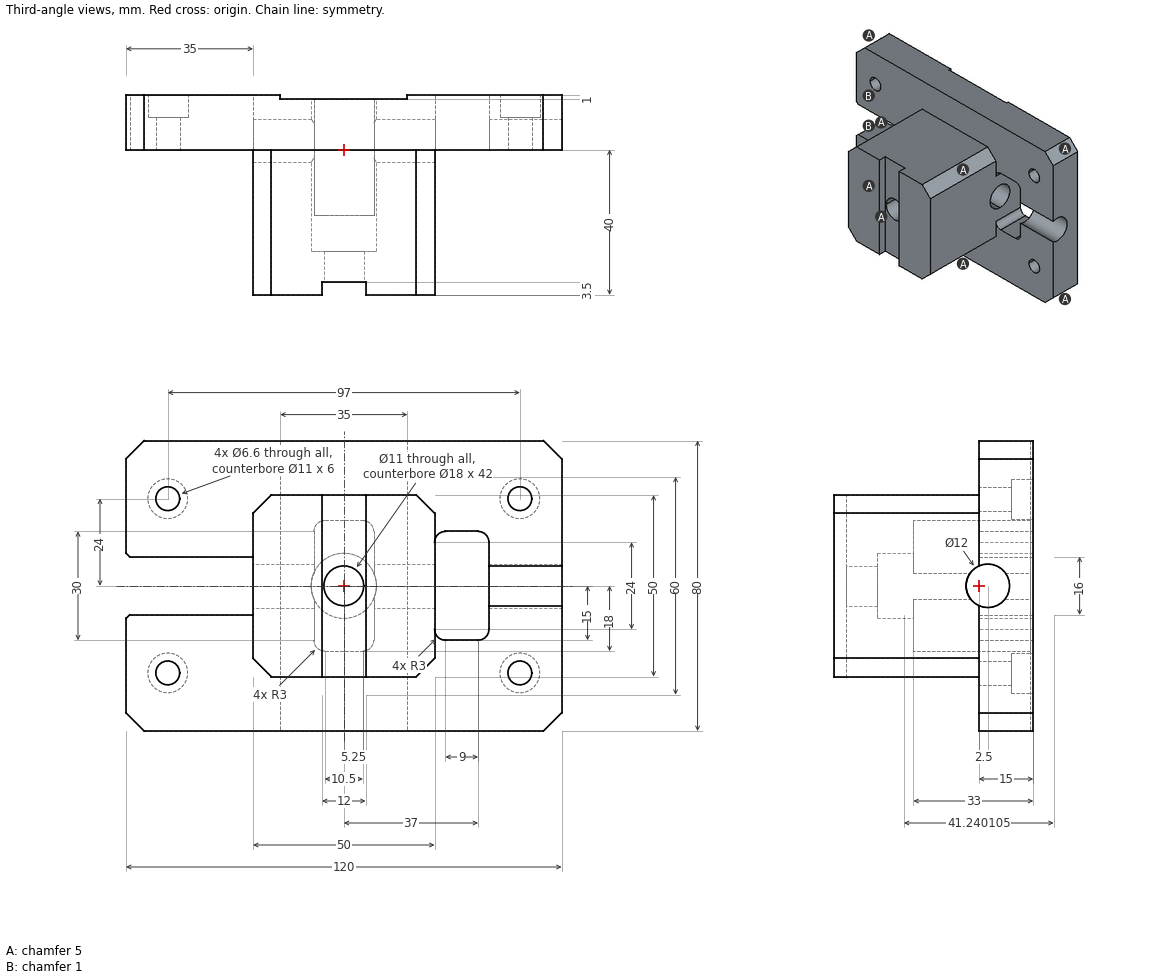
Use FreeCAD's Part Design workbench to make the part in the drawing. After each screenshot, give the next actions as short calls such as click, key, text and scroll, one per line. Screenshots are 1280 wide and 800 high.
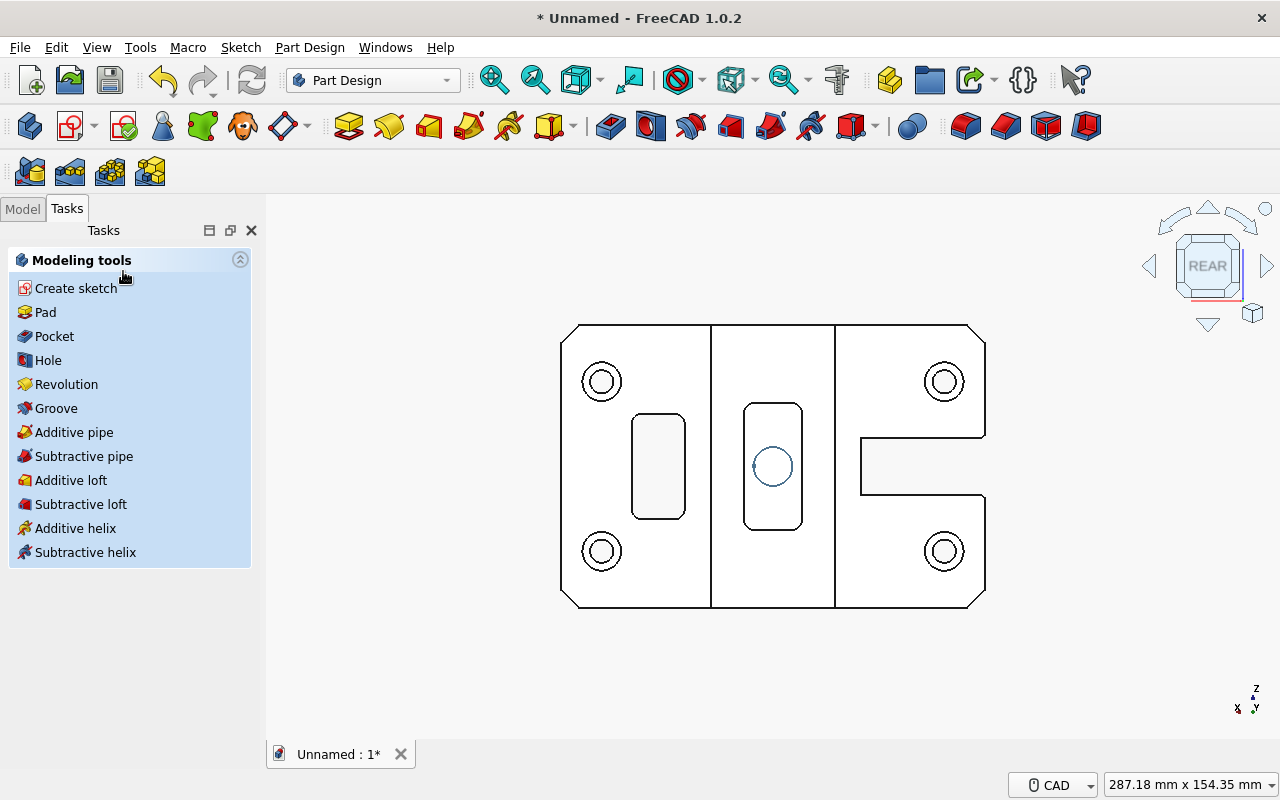
click(652, 126)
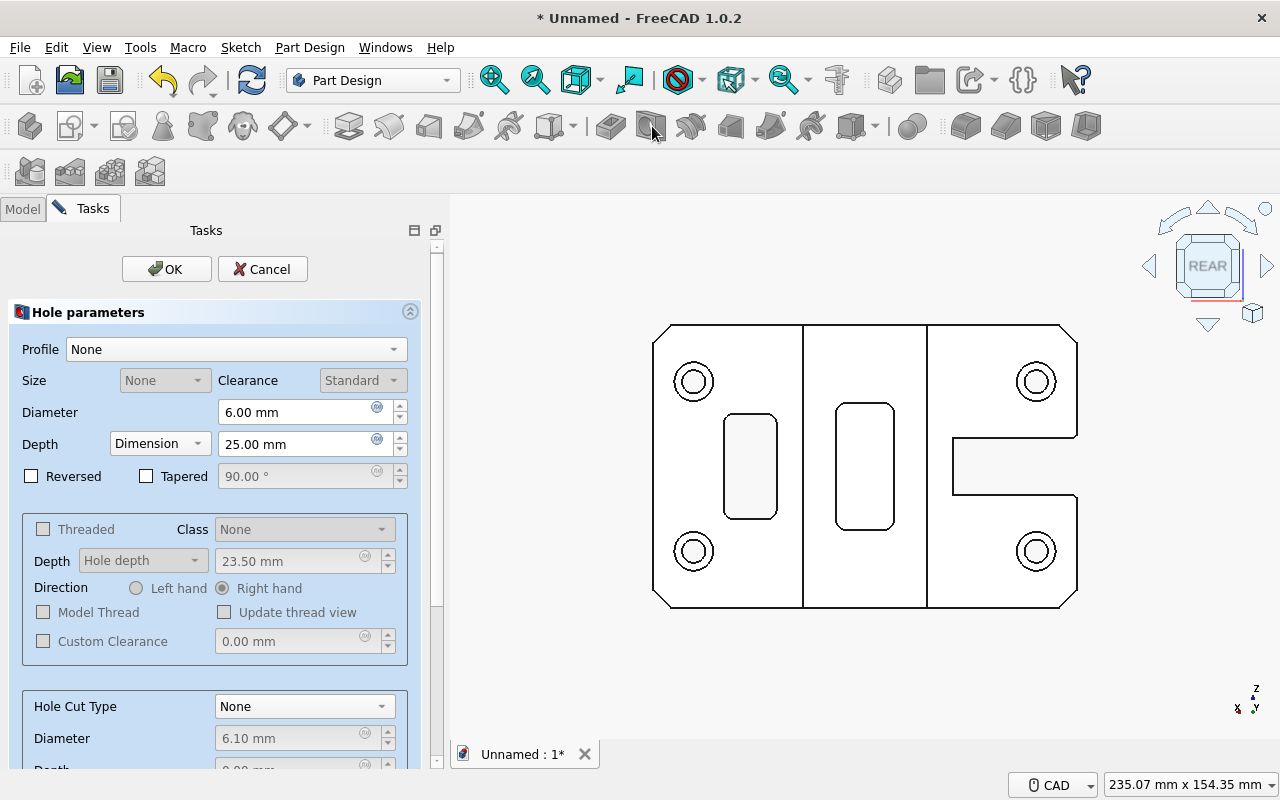
triple_click(305, 412)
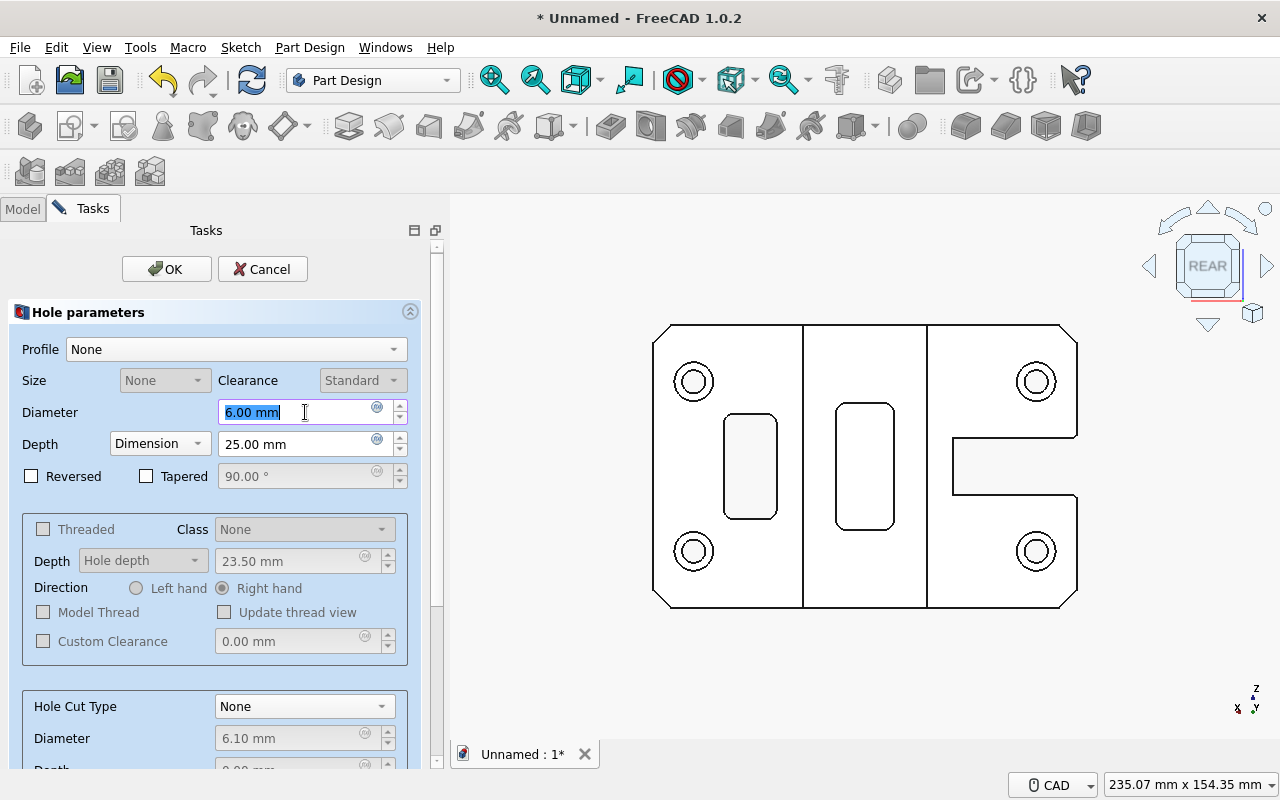
text(11)
key(Tab)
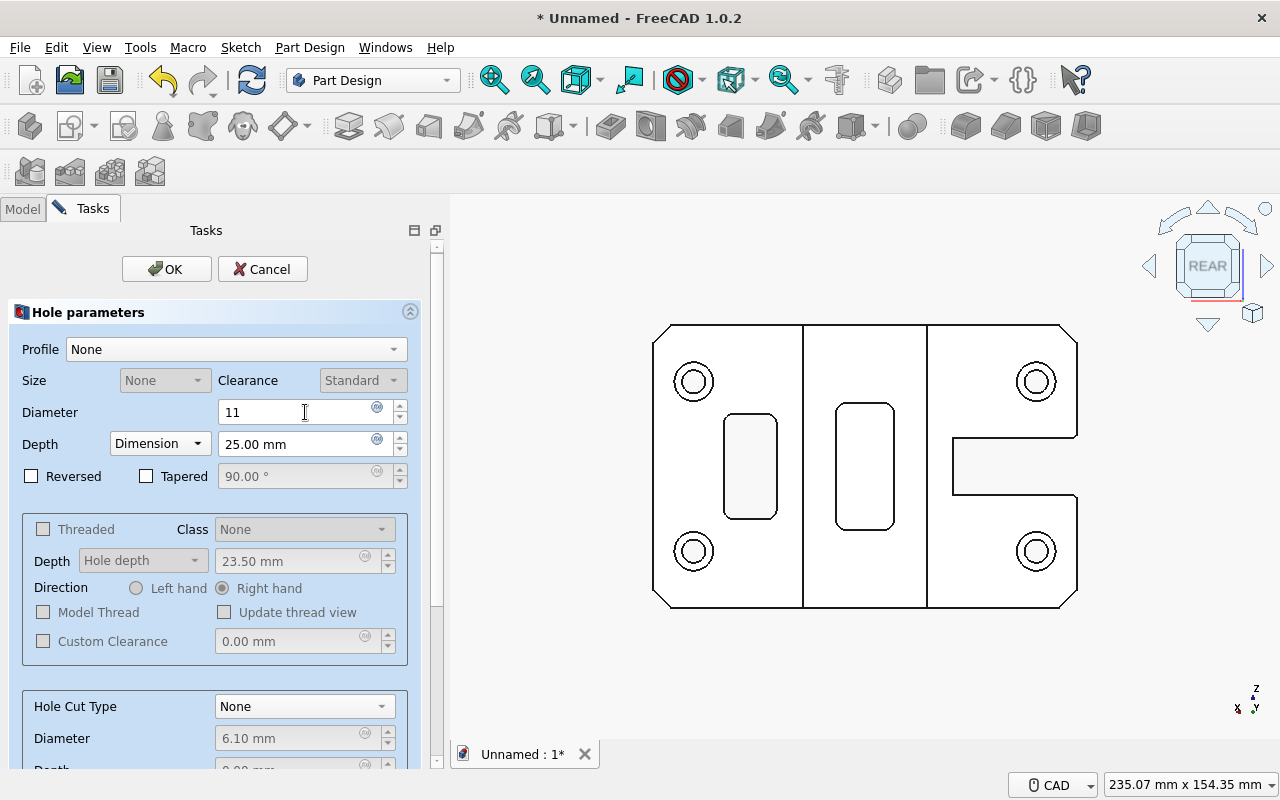
click(161, 444)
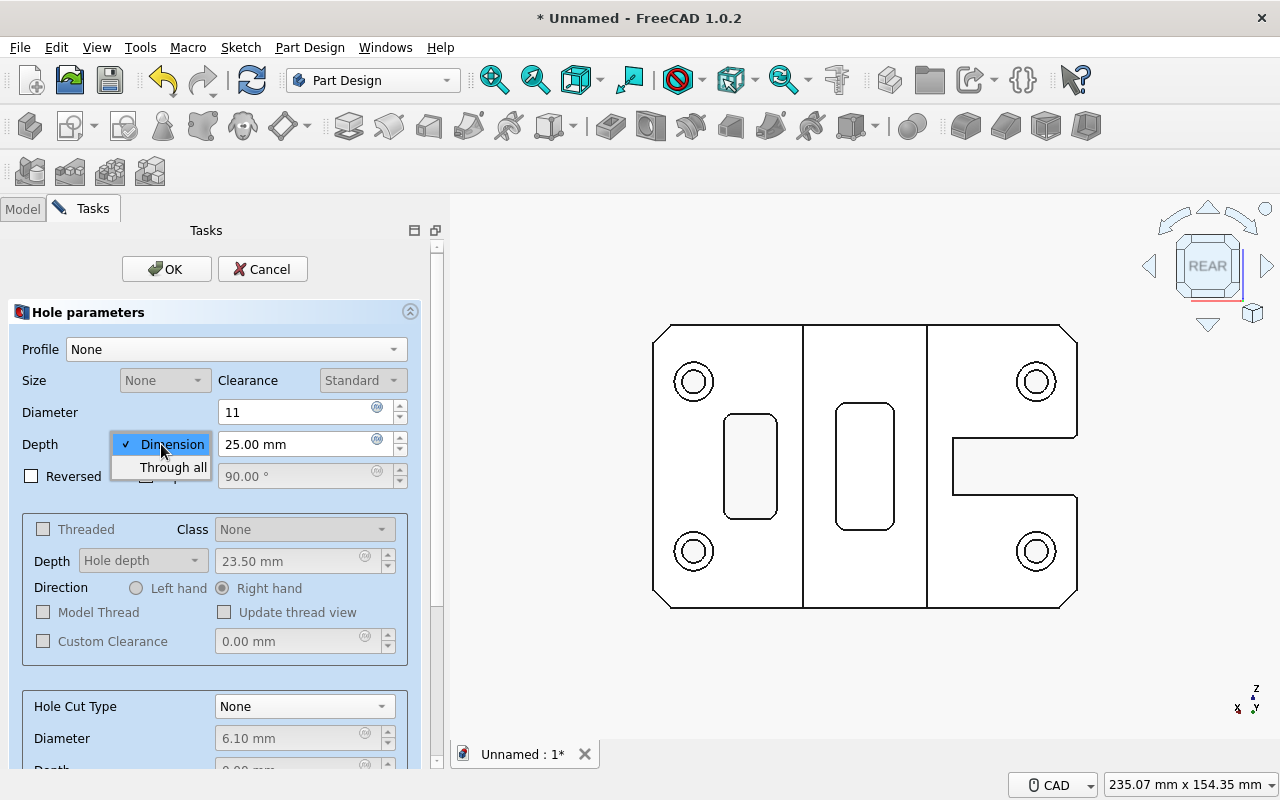
click(160, 468)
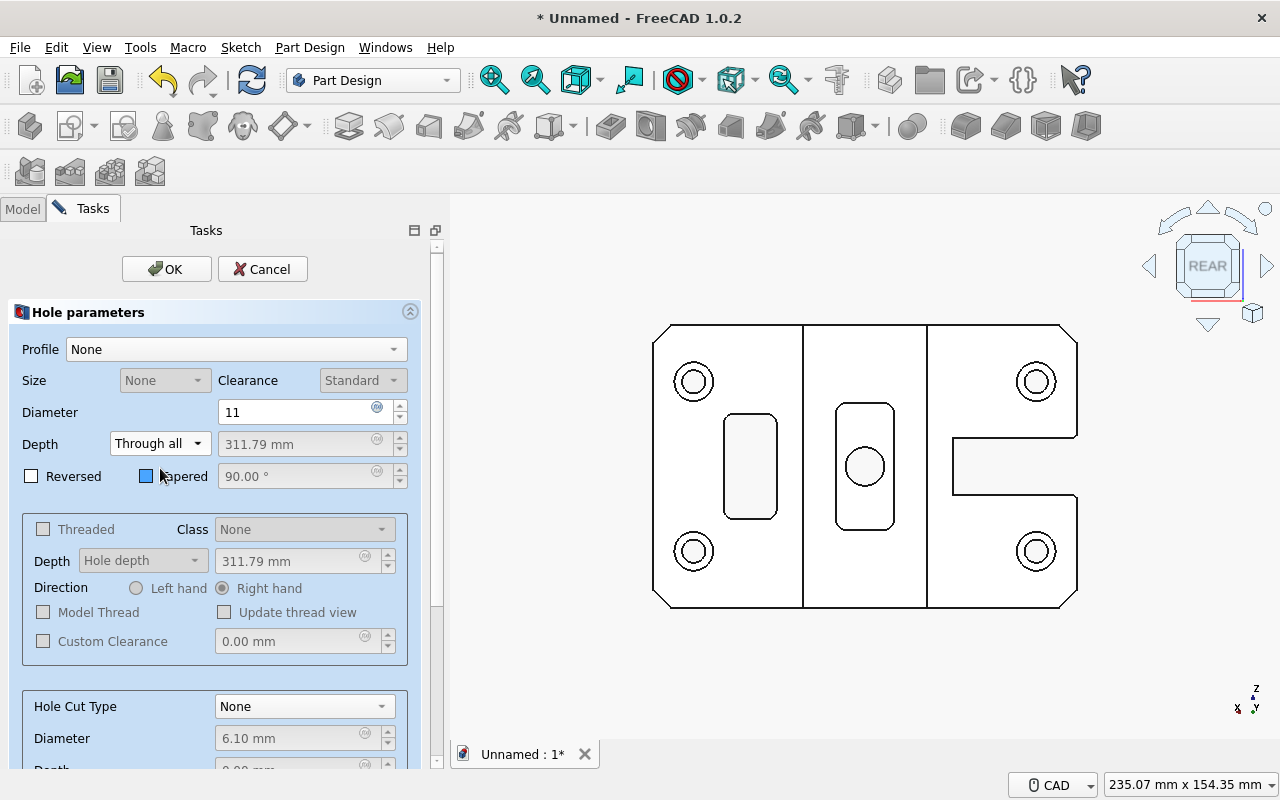
click(306, 706)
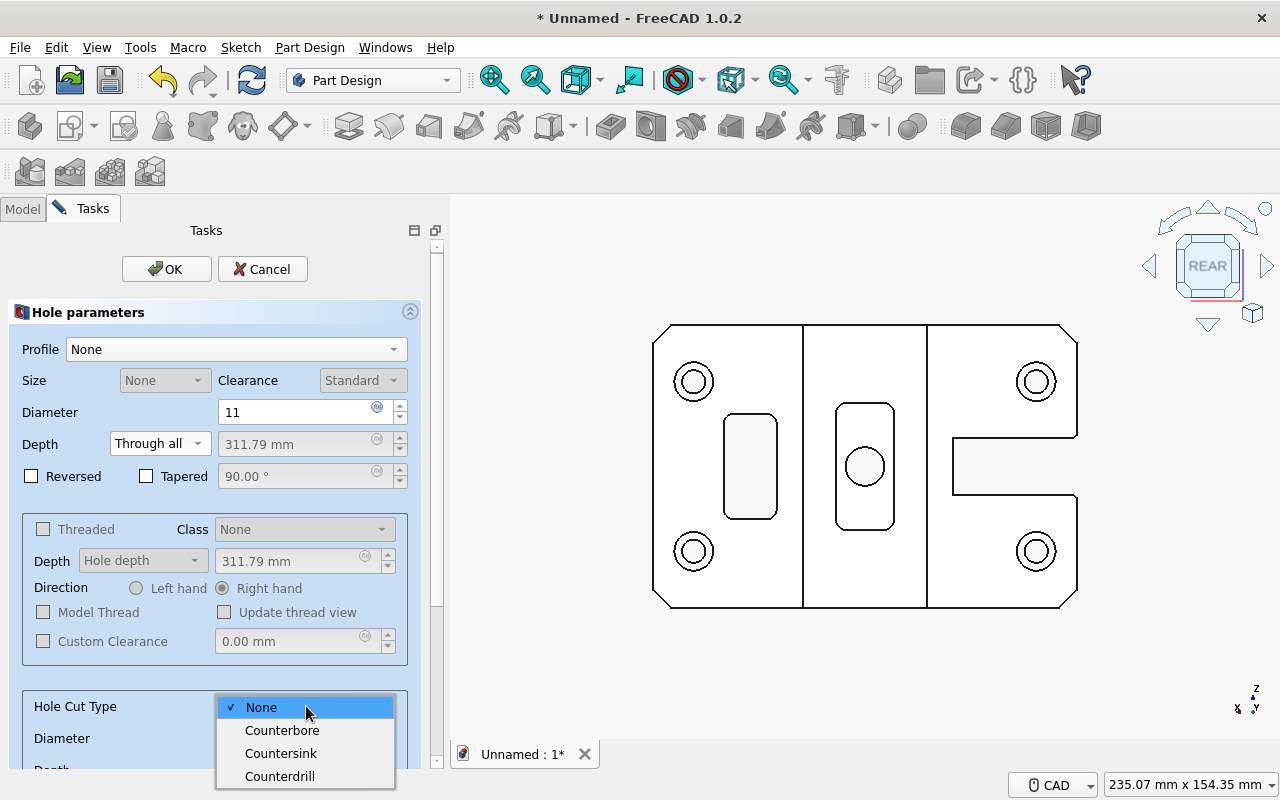
click(304, 730)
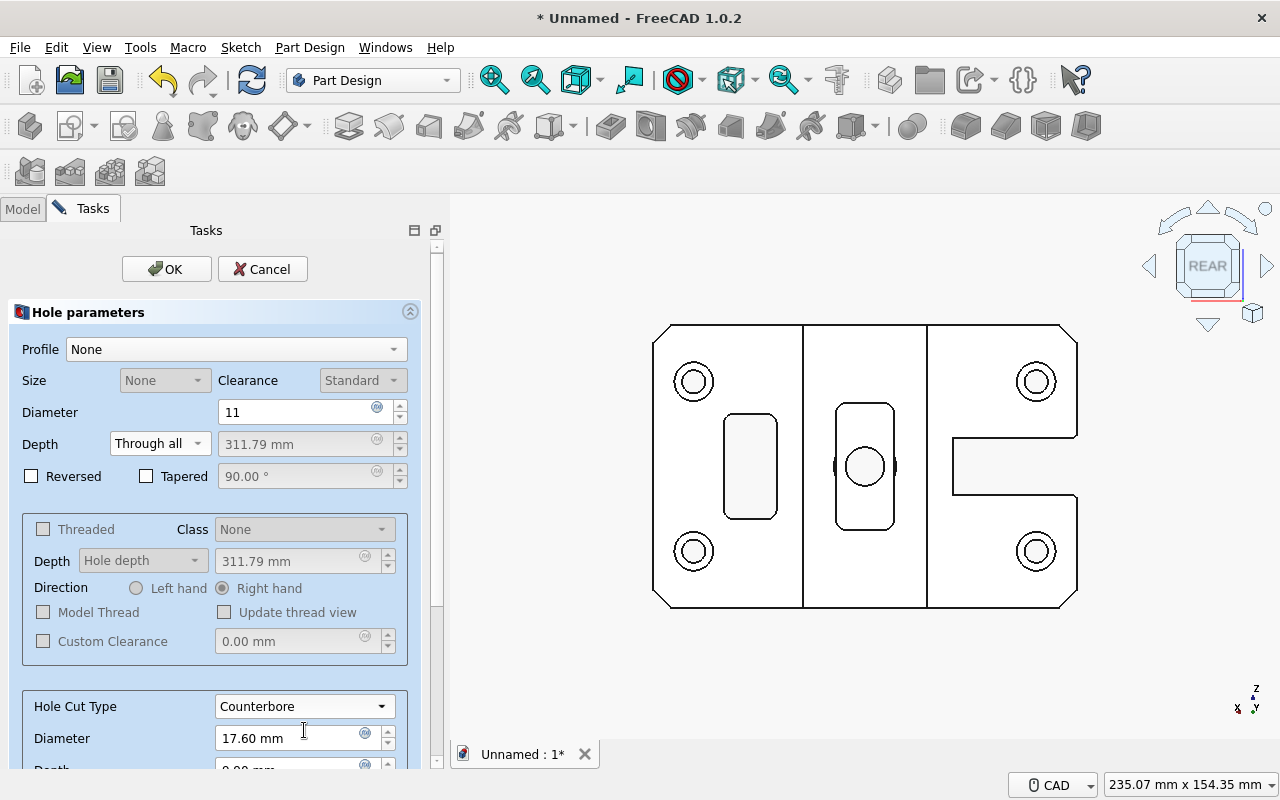
triple_click(298, 738)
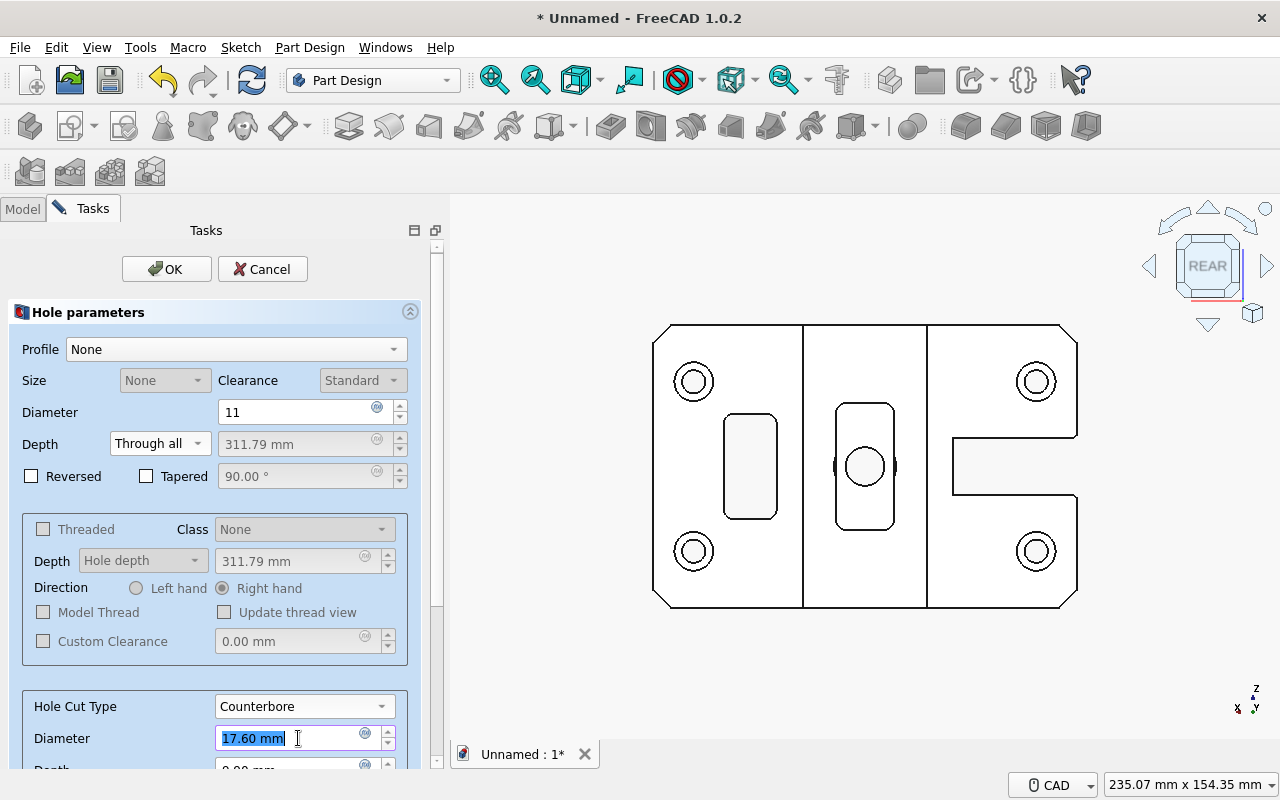
text(18)
key(Tab)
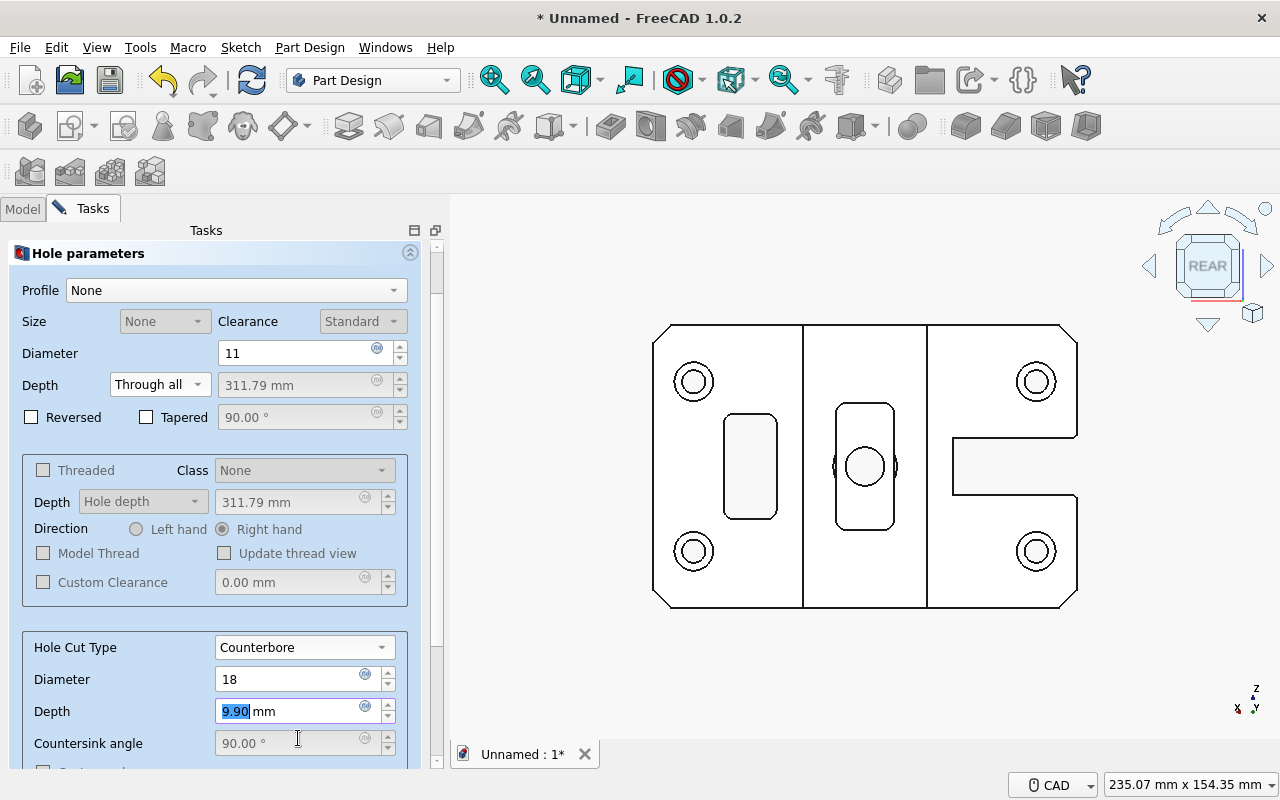
text(42)
key(Tab)